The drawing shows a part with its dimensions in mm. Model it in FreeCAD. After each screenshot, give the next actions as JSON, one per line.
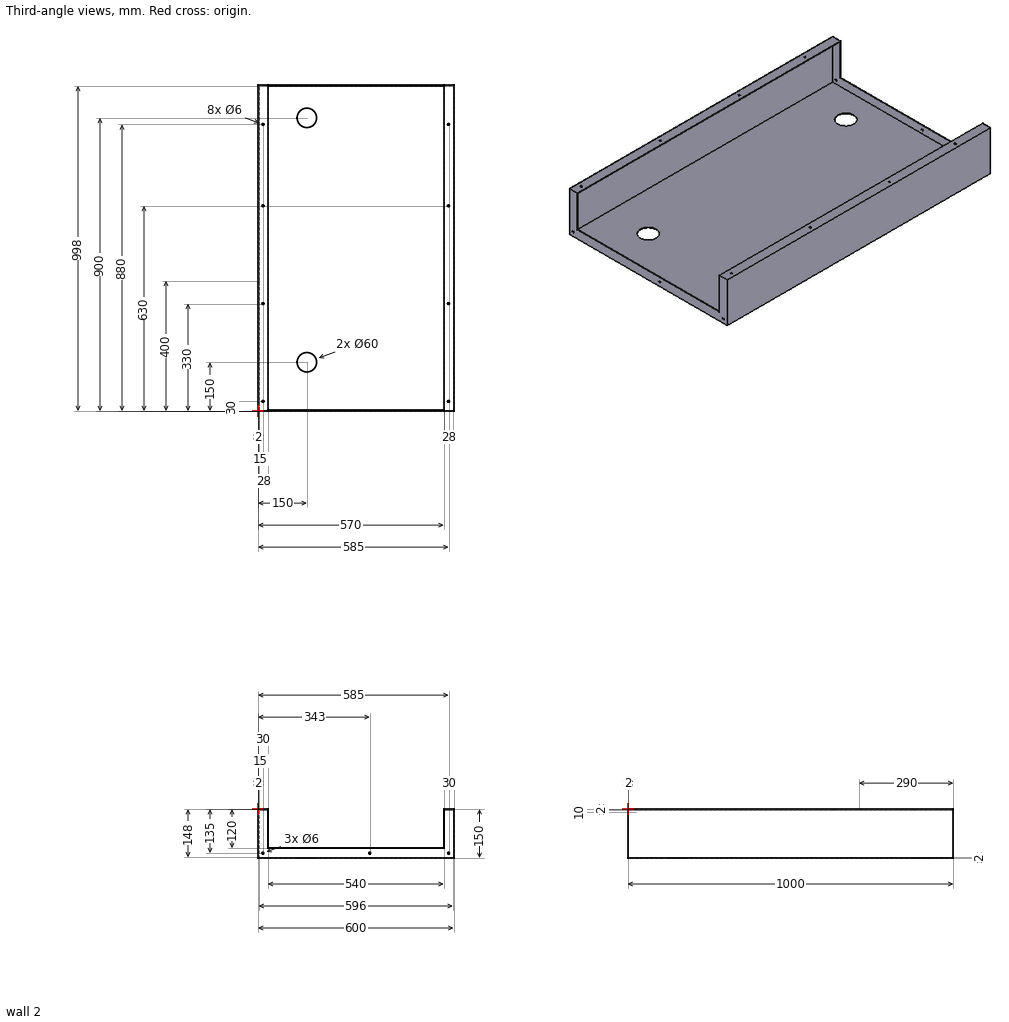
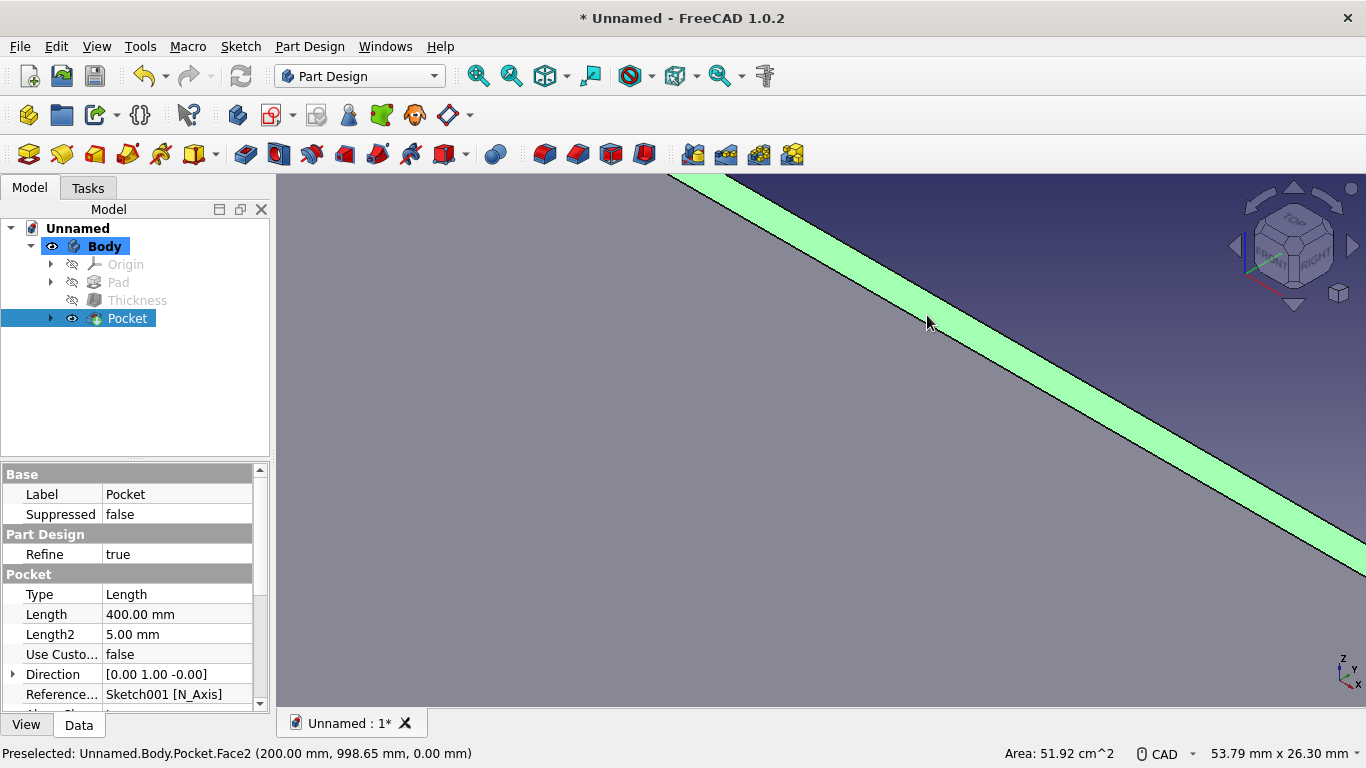
{"action": "left_click", "coordinate": [270, 116]}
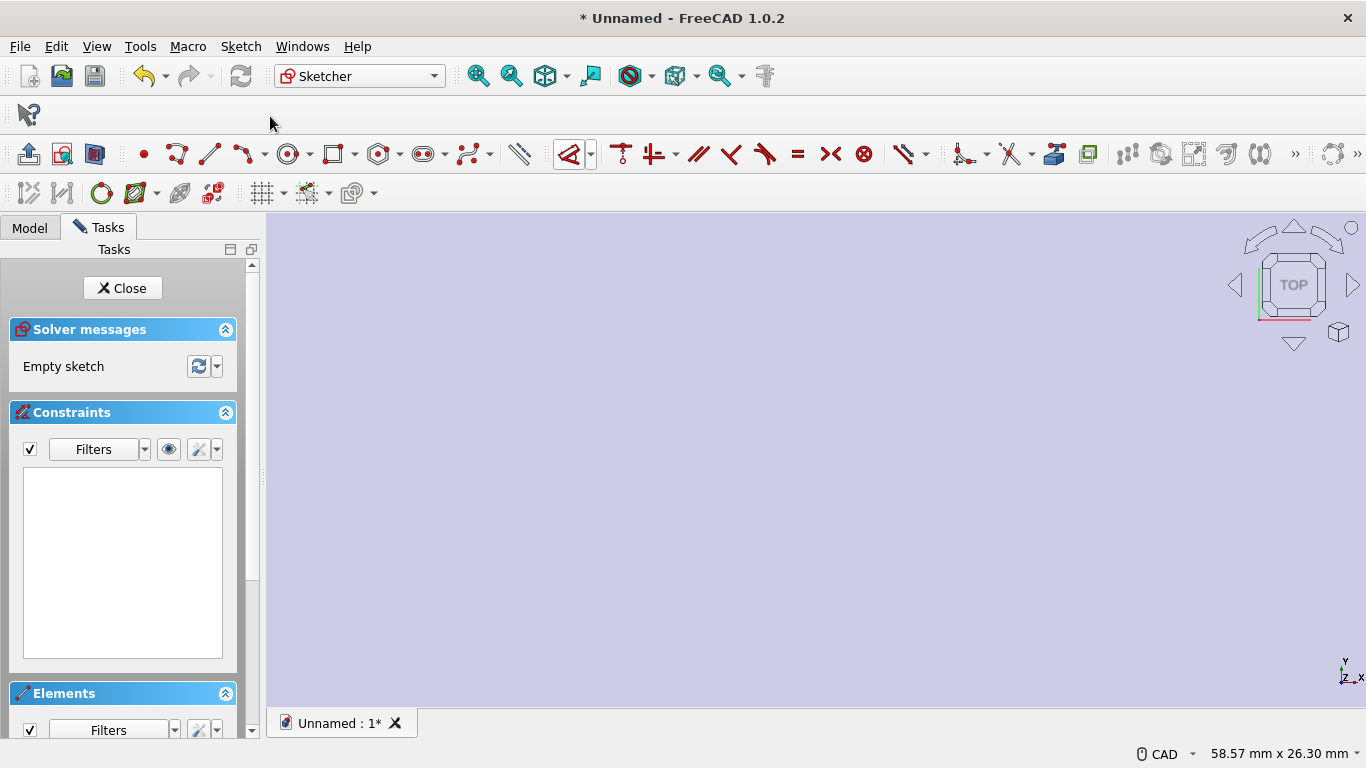
{"action": "scroll", "coordinate": [748, 460], "scroll_direction": "down", "scroll_amount": 15}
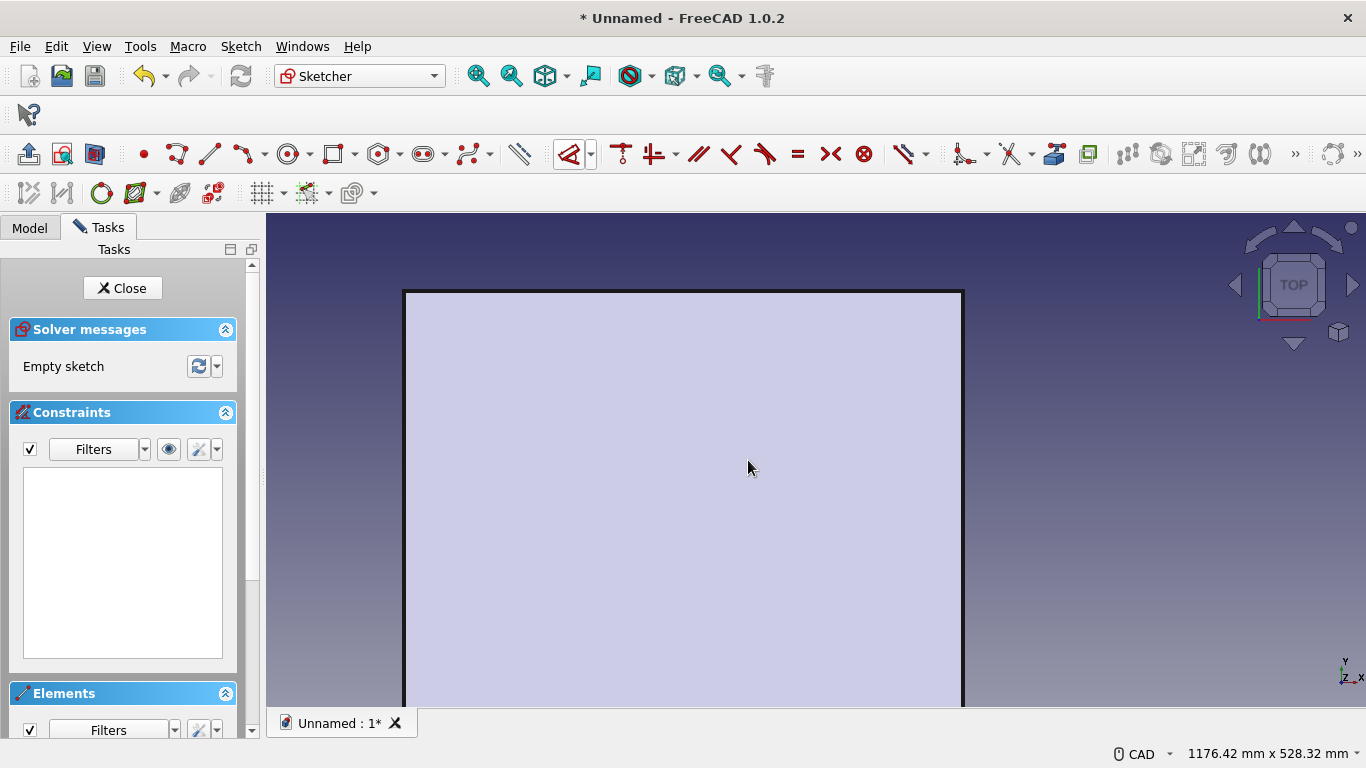
{"action": "scroll", "coordinate": [776, 331], "scroll_direction": "down", "scroll_amount": 6}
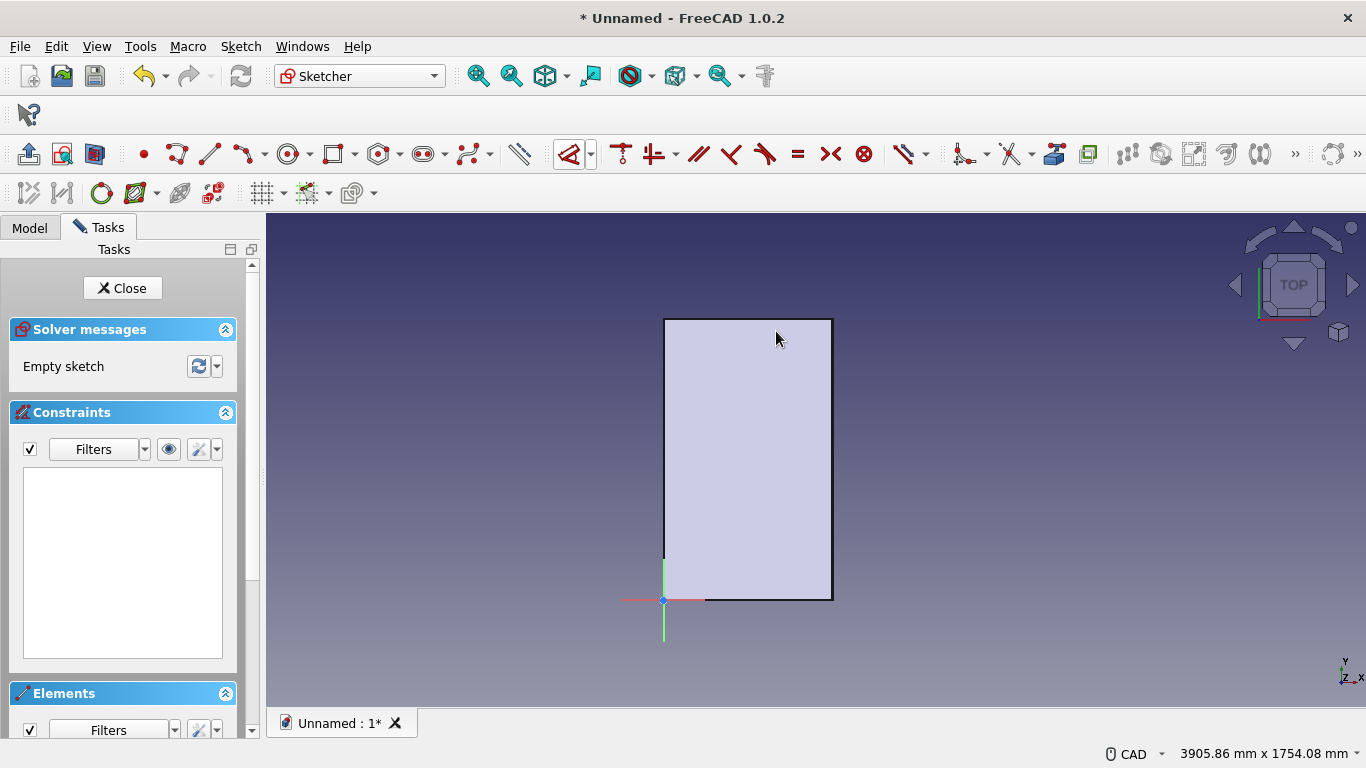
{"action": "left_click", "coordinate": [332, 154]}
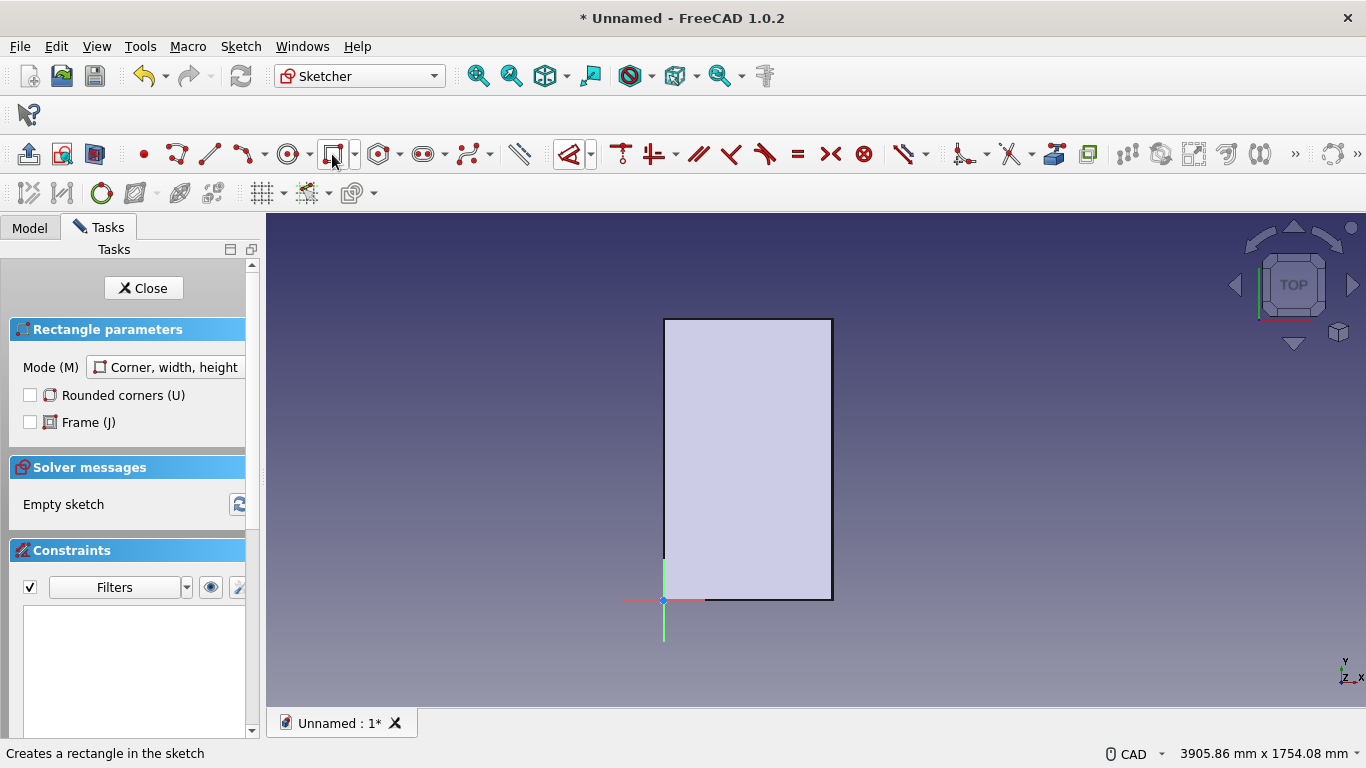
{"action": "scroll", "coordinate": [664, 319], "scroll_direction": "up", "scroll_amount": 17}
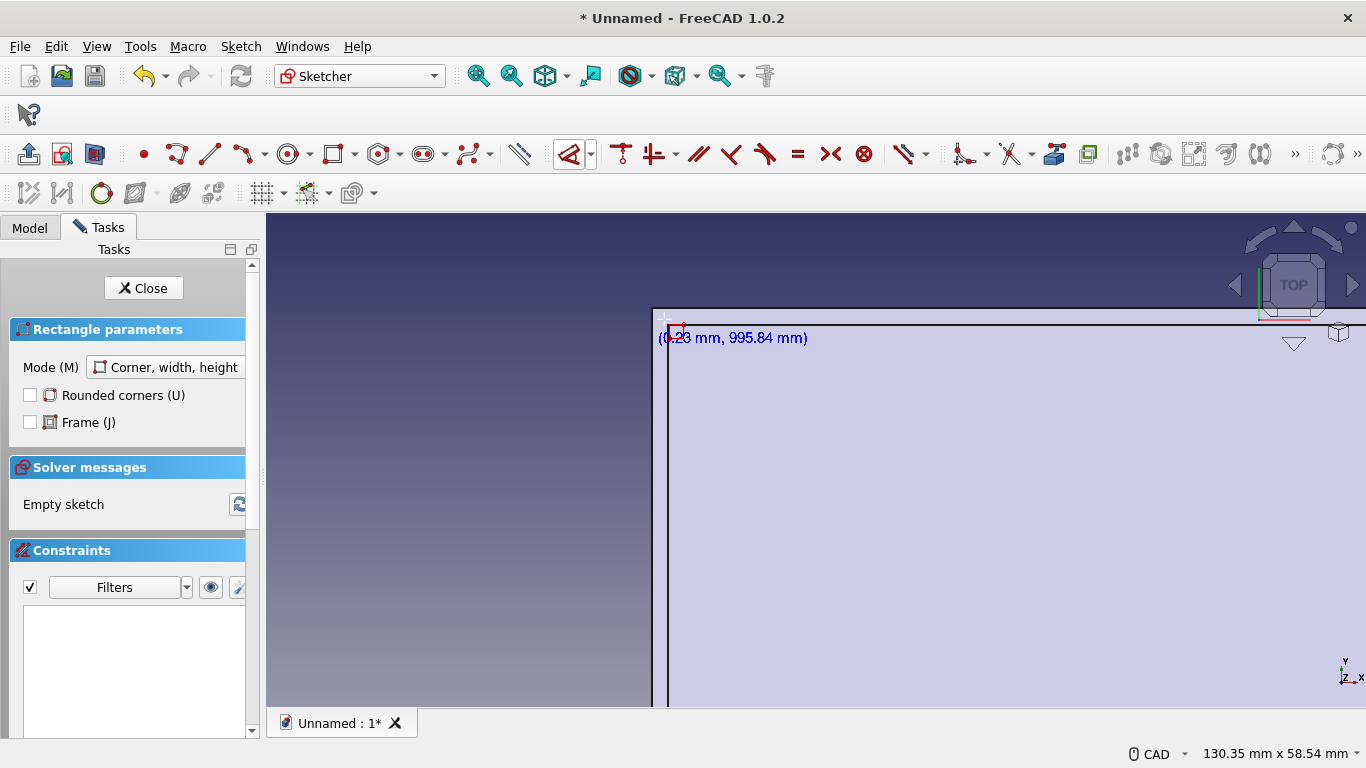
{"action": "left_click", "coordinate": [668, 325]}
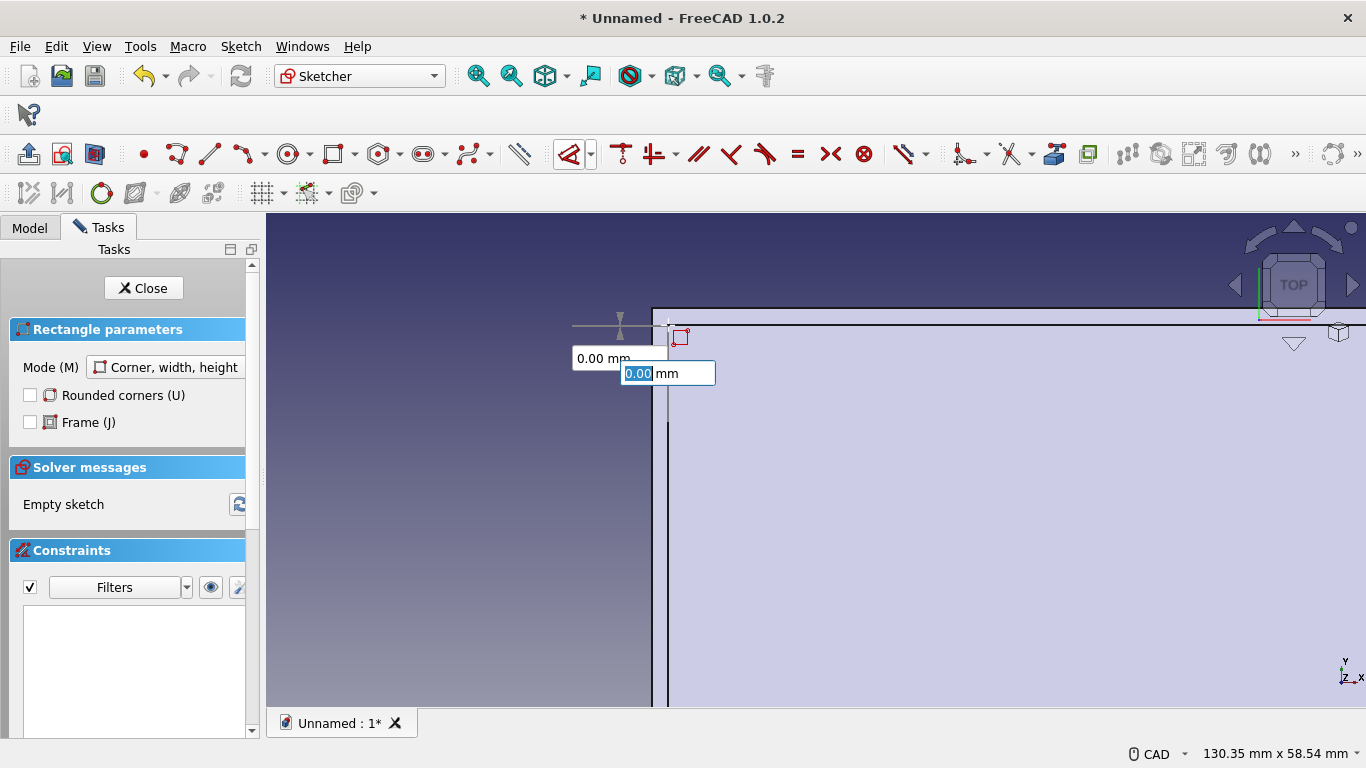
{"action": "scroll", "coordinate": [644, 287], "scroll_direction": "down", "scroll_amount": 16}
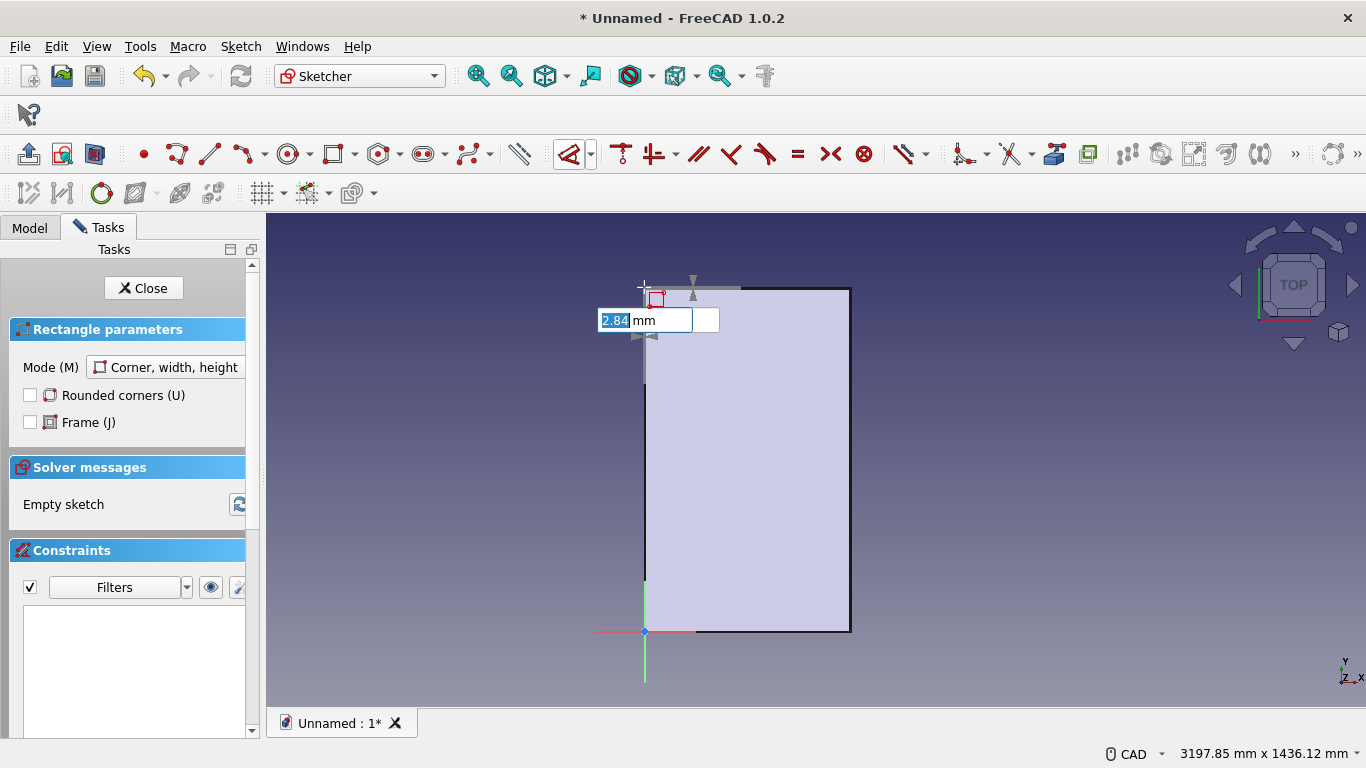
{"action": "scroll", "coordinate": [655, 632], "scroll_direction": "up", "scroll_amount": 3}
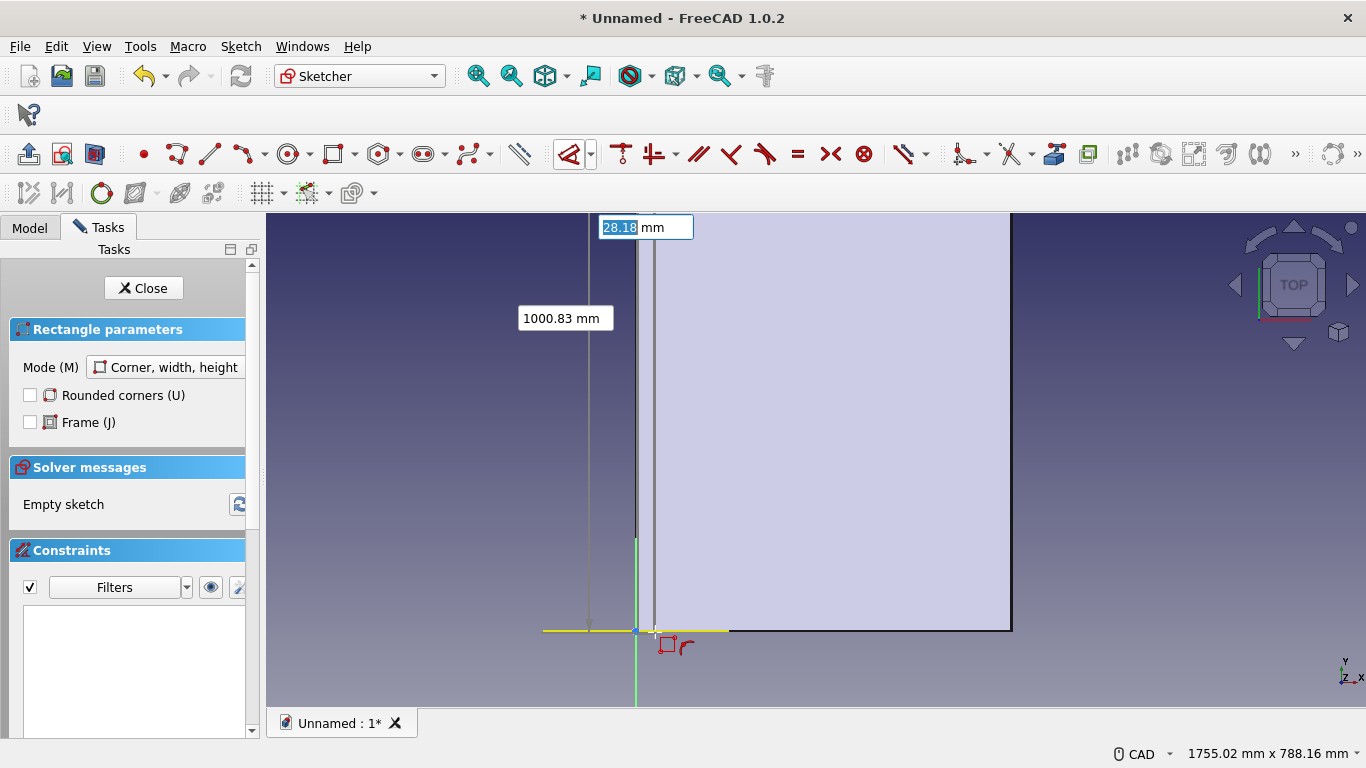
{"action": "left_click", "coordinate": [655, 631]}